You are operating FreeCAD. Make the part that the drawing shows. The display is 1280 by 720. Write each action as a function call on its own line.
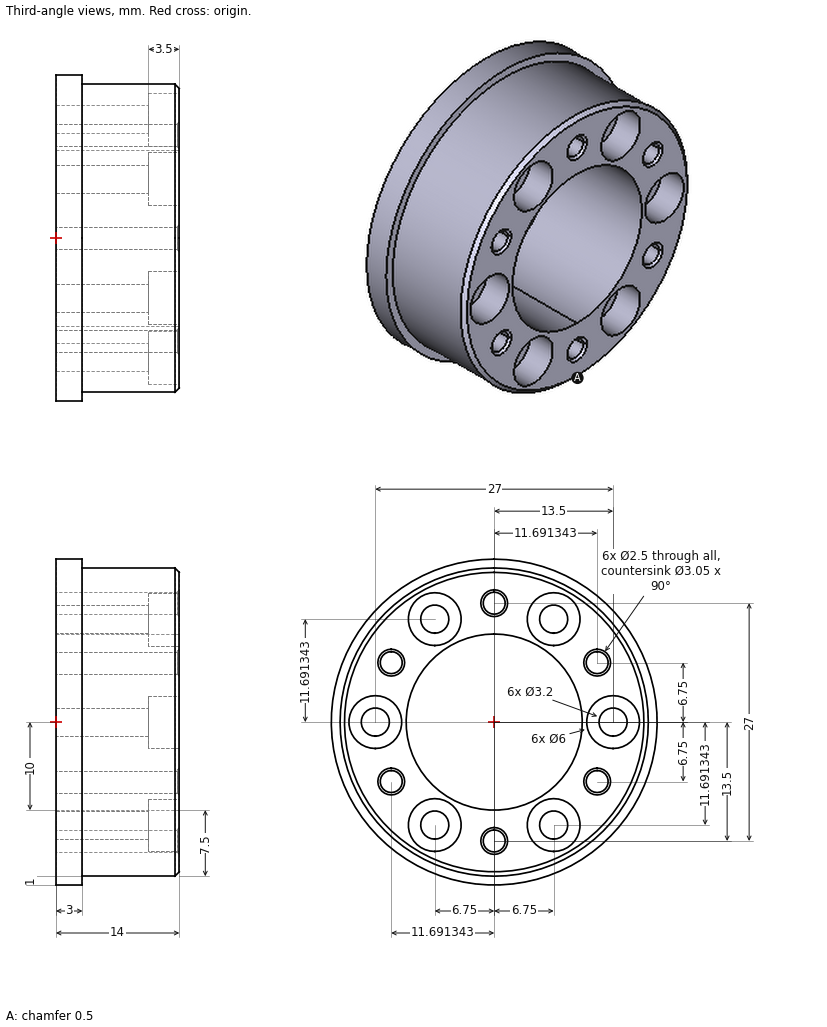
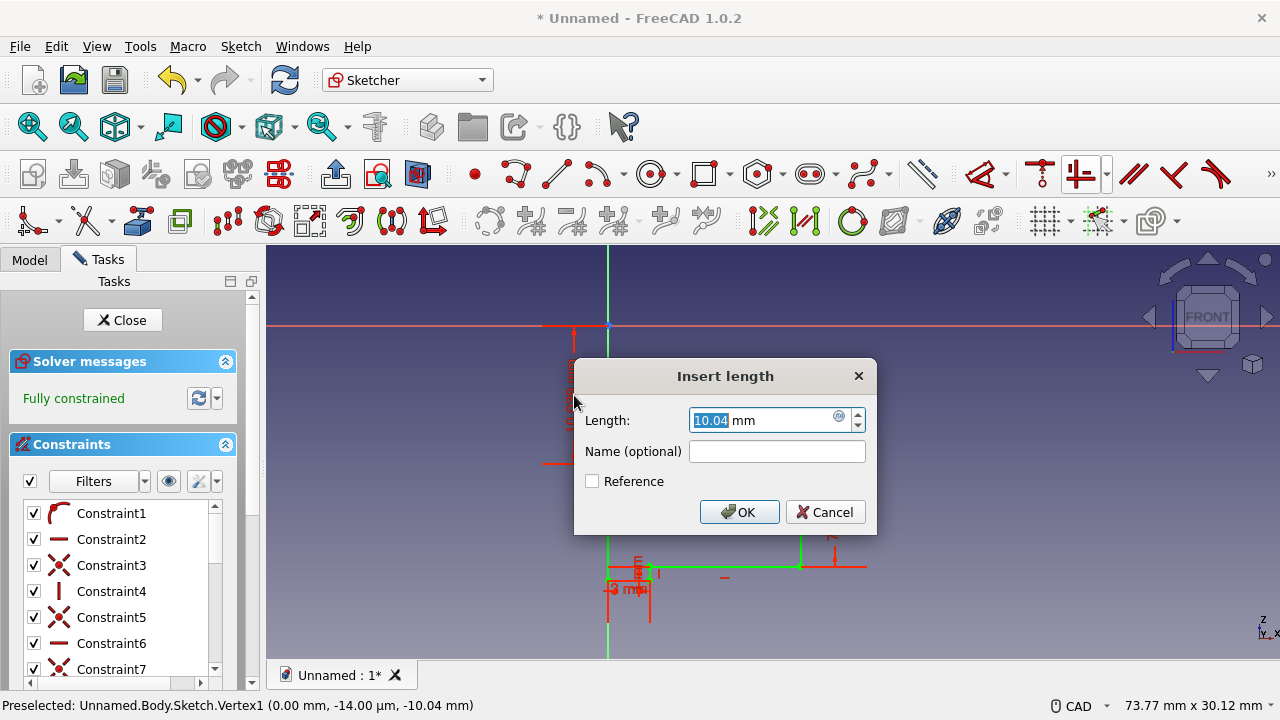
text(10)
key(Return)
key(Escape)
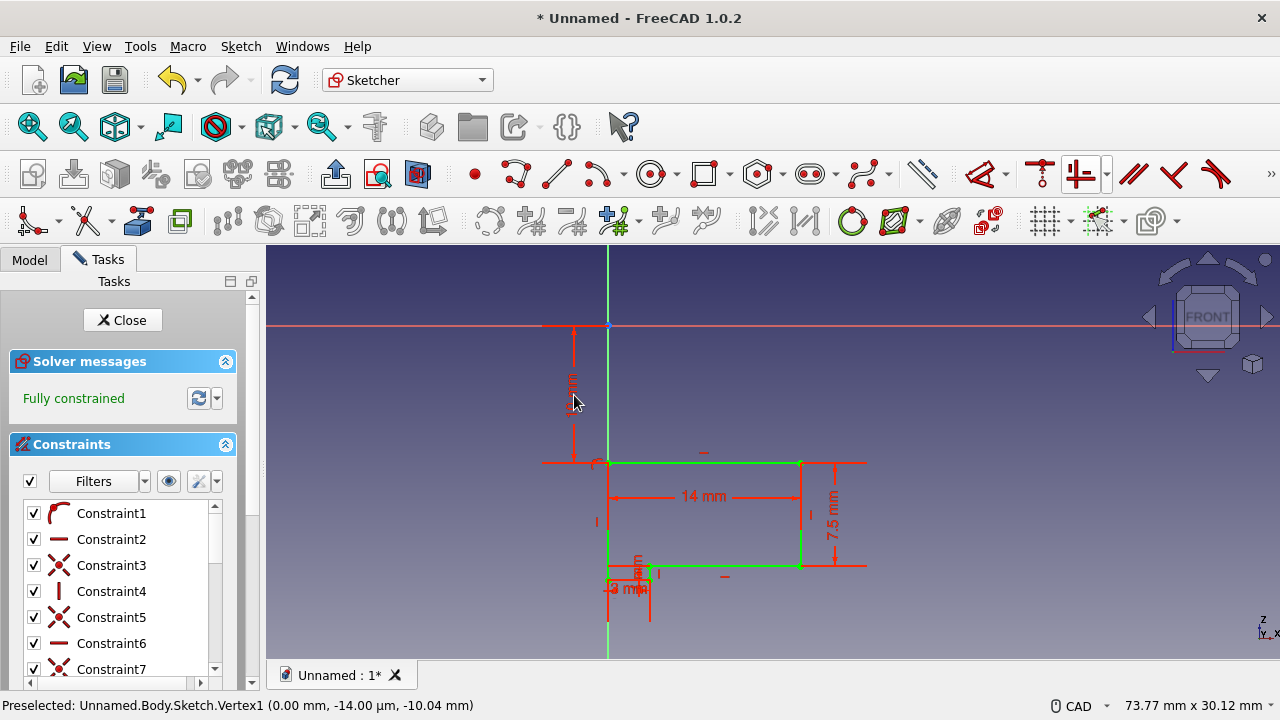
click(123, 320)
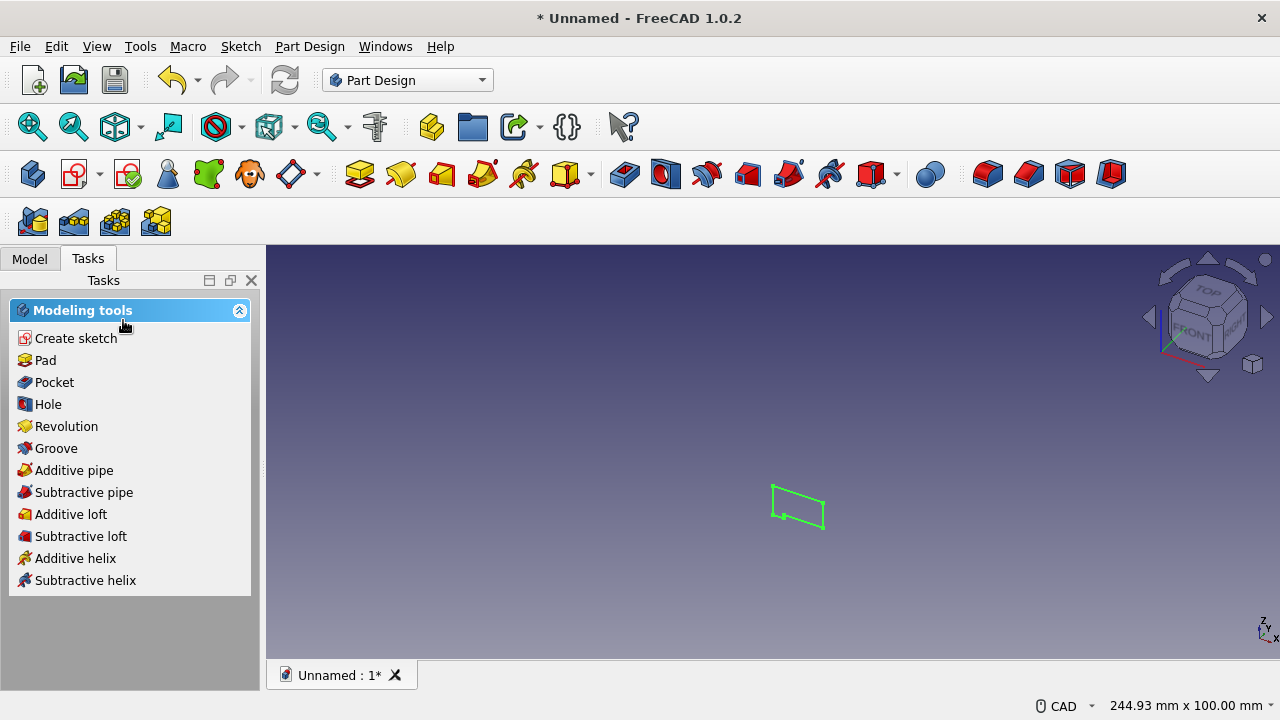
click(401, 174)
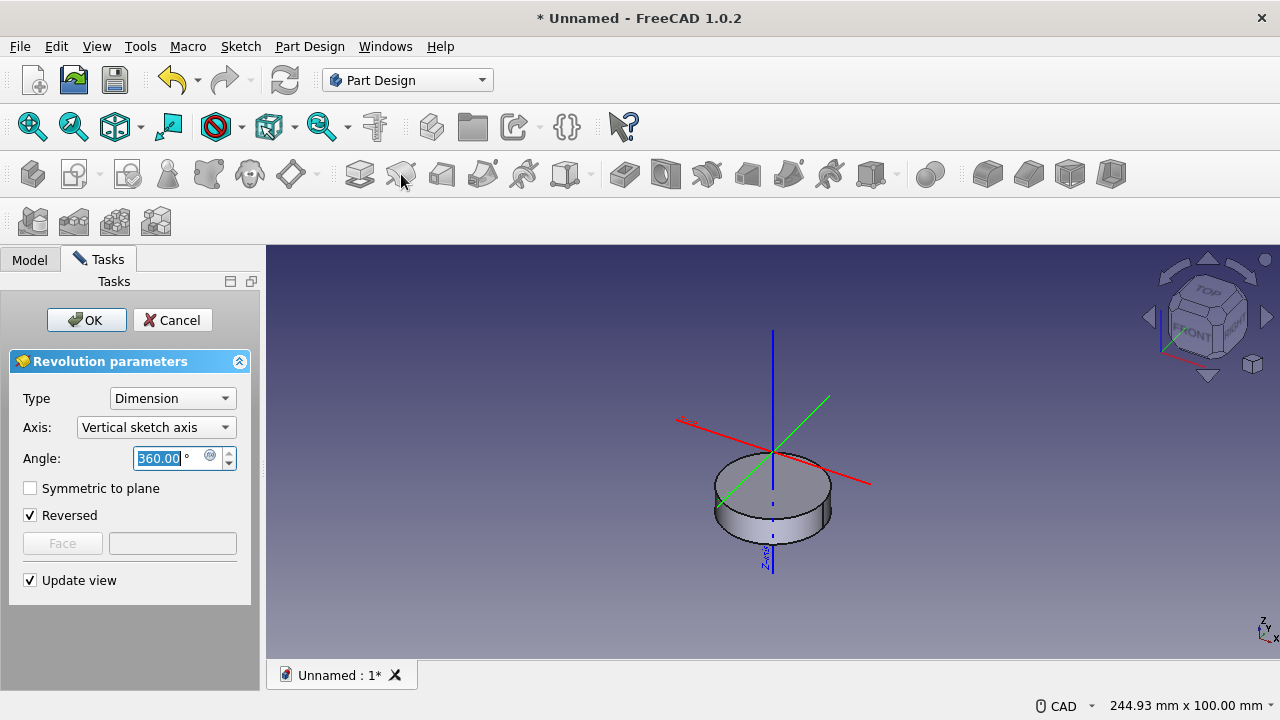
click(157, 428)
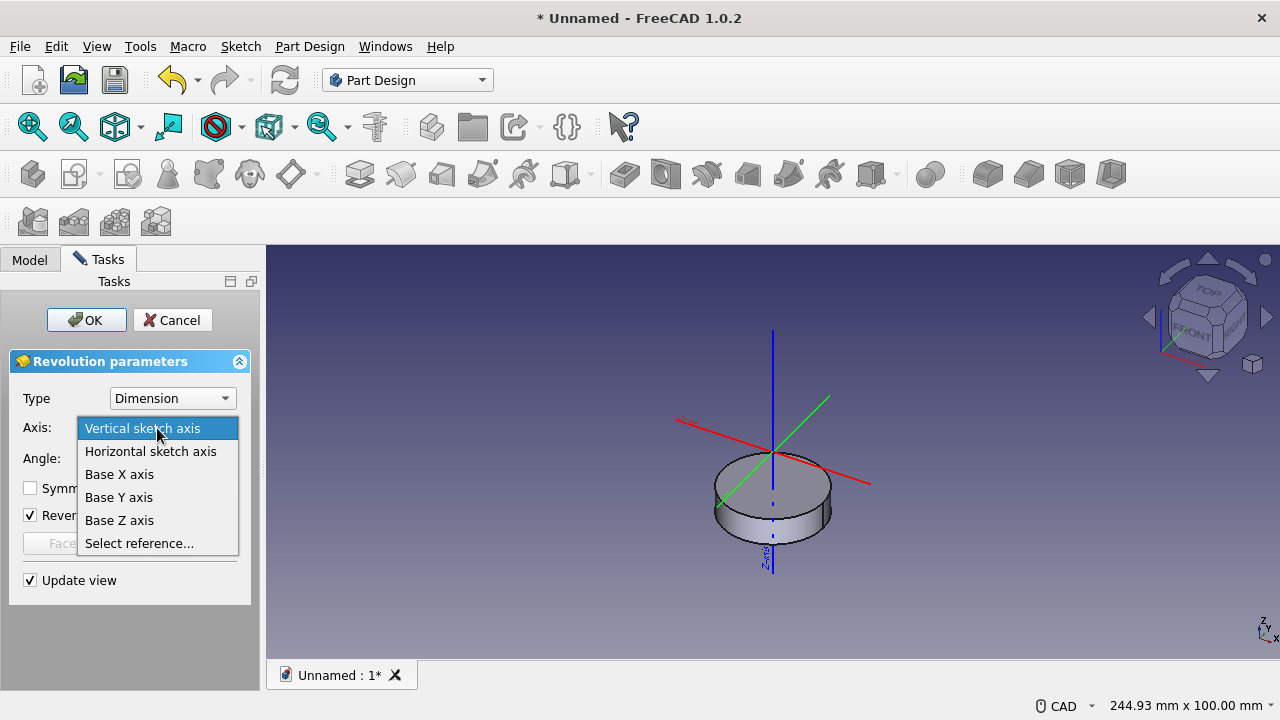
click(156, 452)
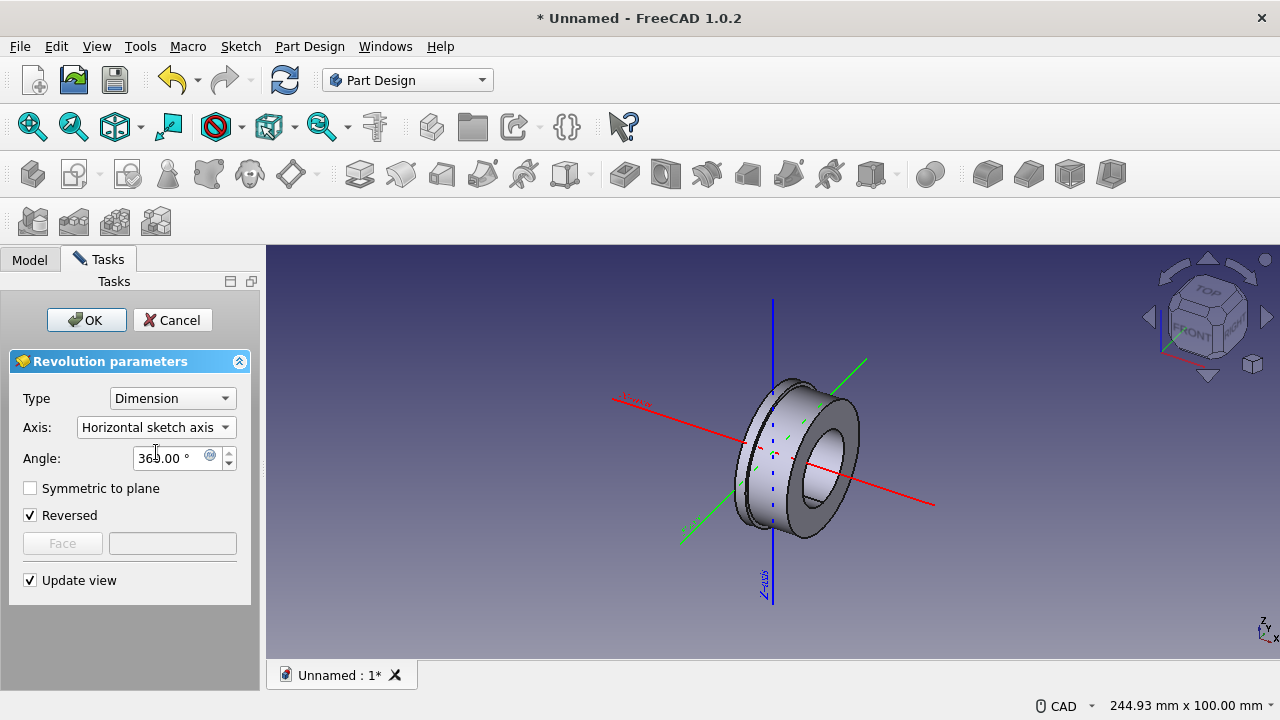
click(87, 320)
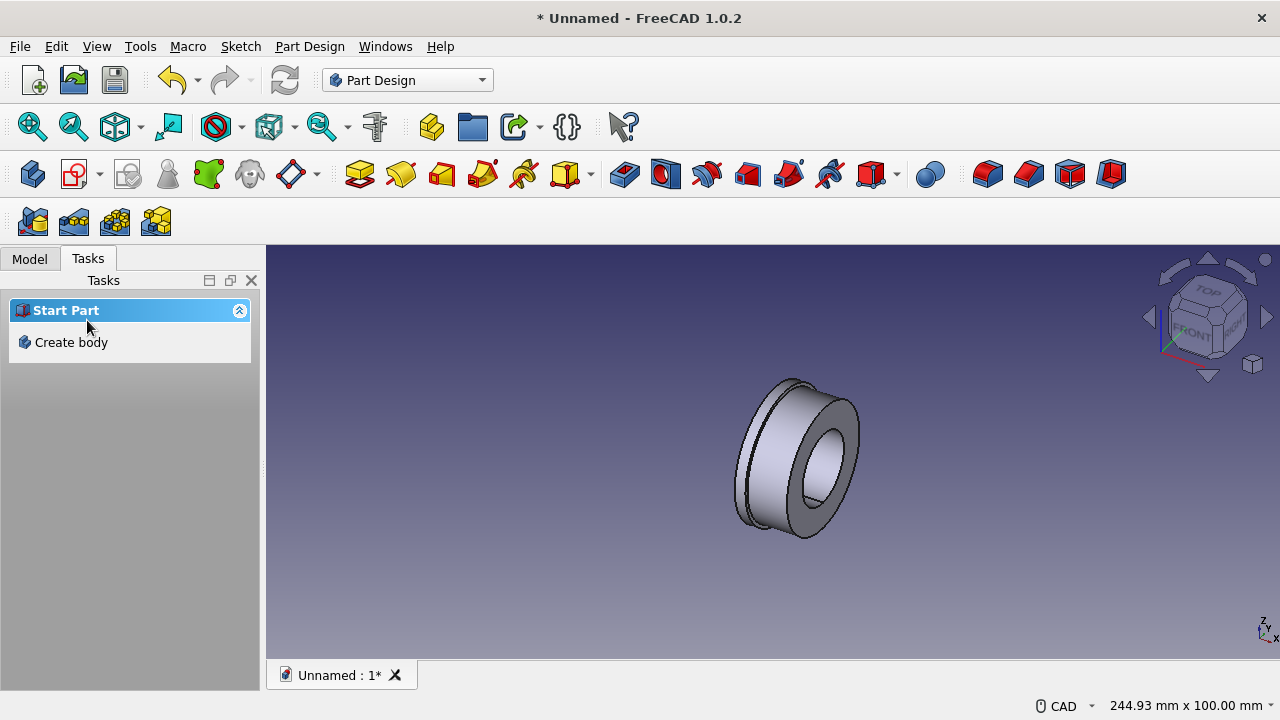
click(844, 413)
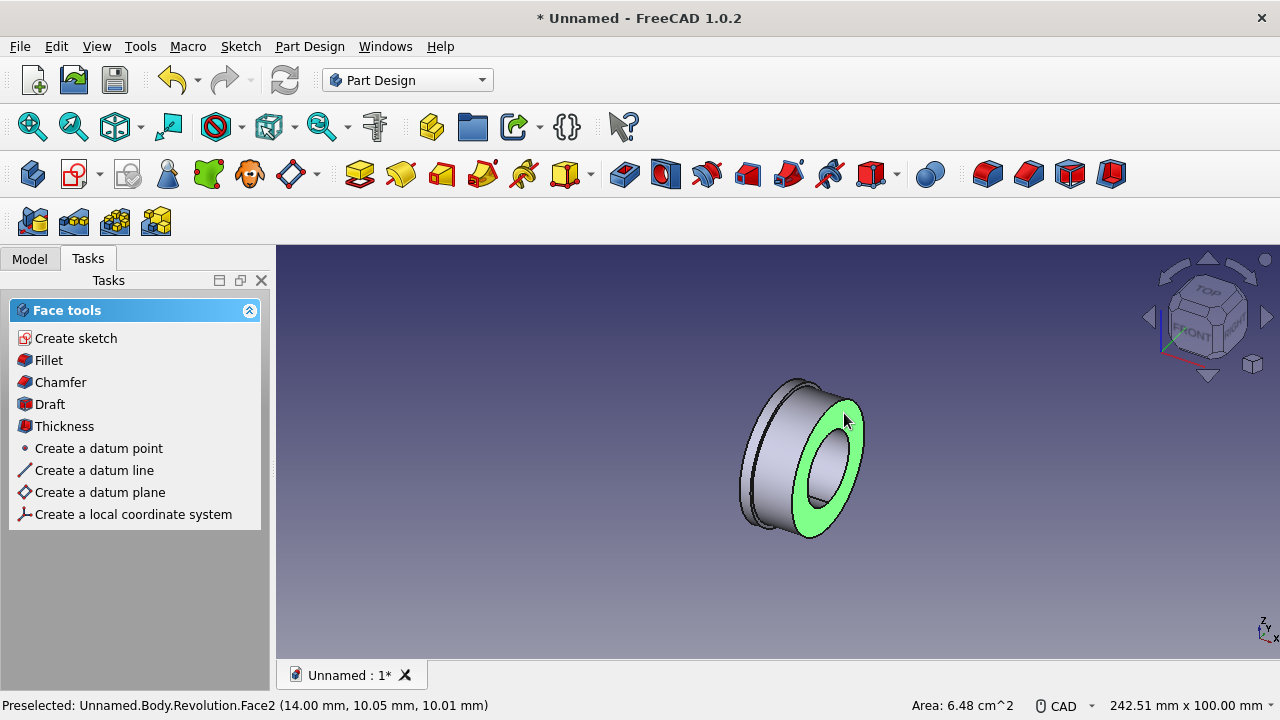
click(74, 174)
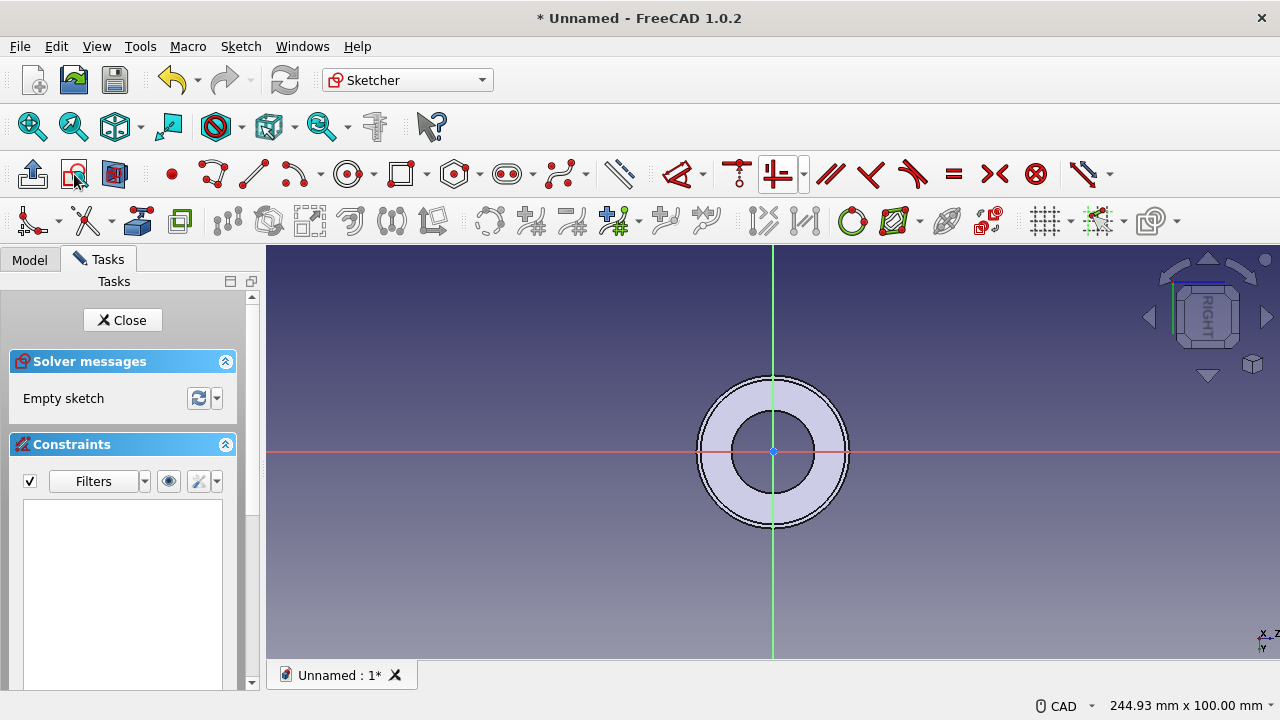
scroll(829, 452, up, 4)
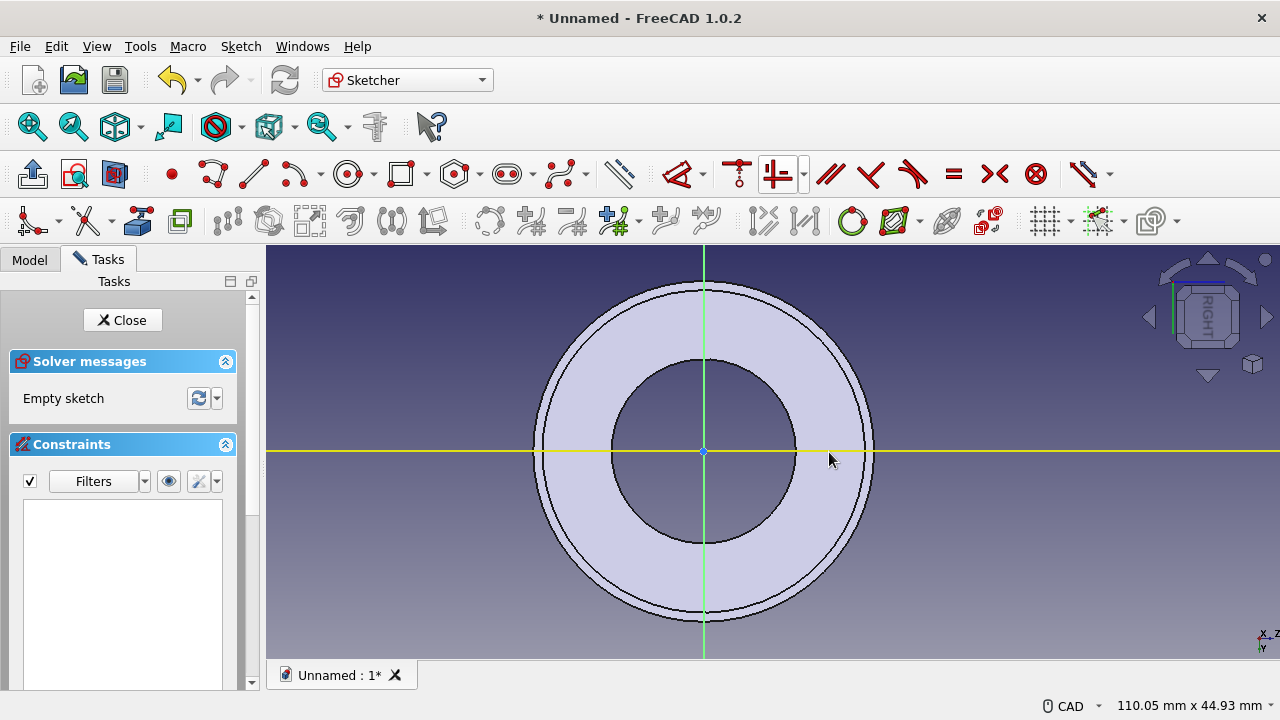
click(348, 174)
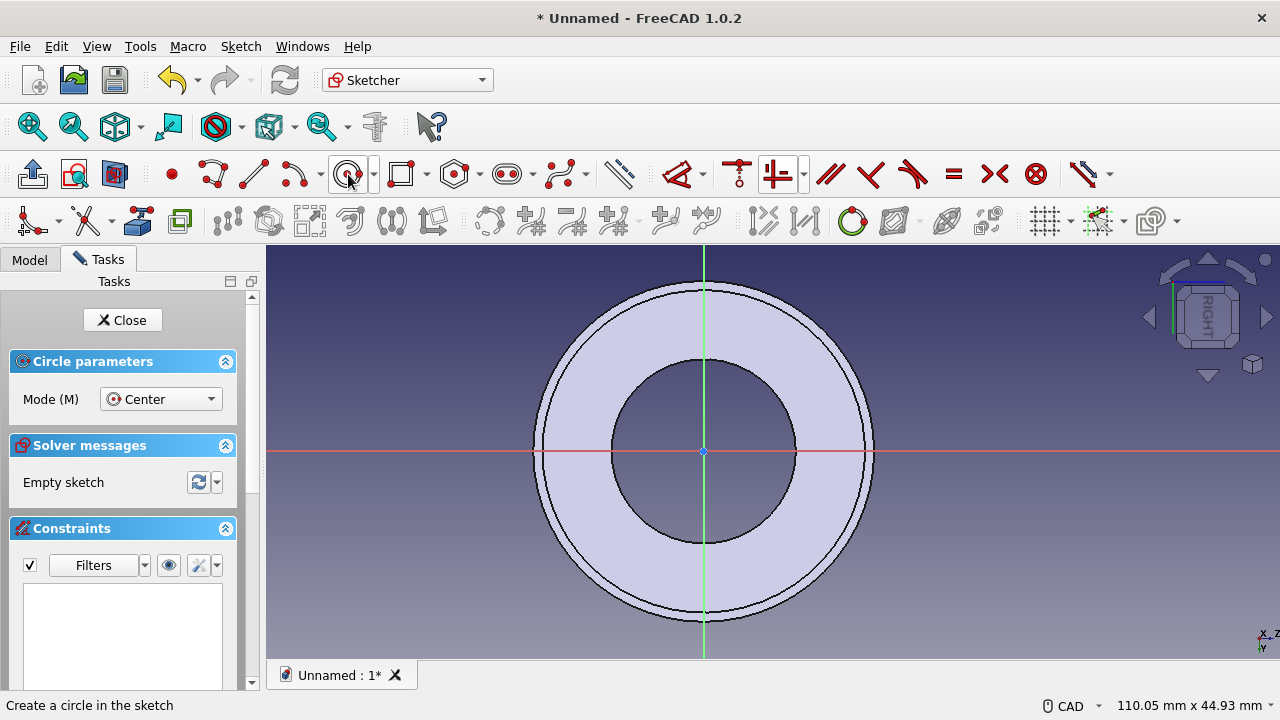
scroll(704, 576, up, 3)